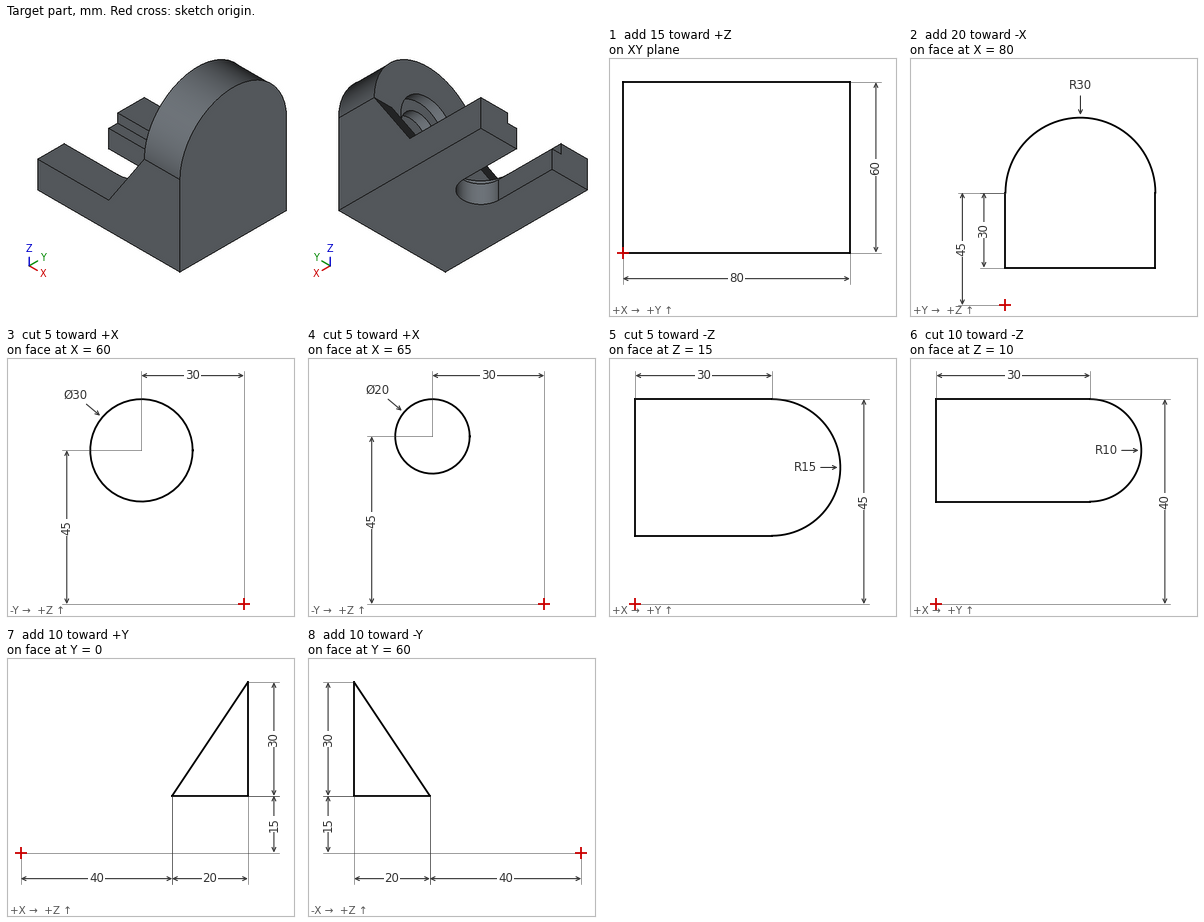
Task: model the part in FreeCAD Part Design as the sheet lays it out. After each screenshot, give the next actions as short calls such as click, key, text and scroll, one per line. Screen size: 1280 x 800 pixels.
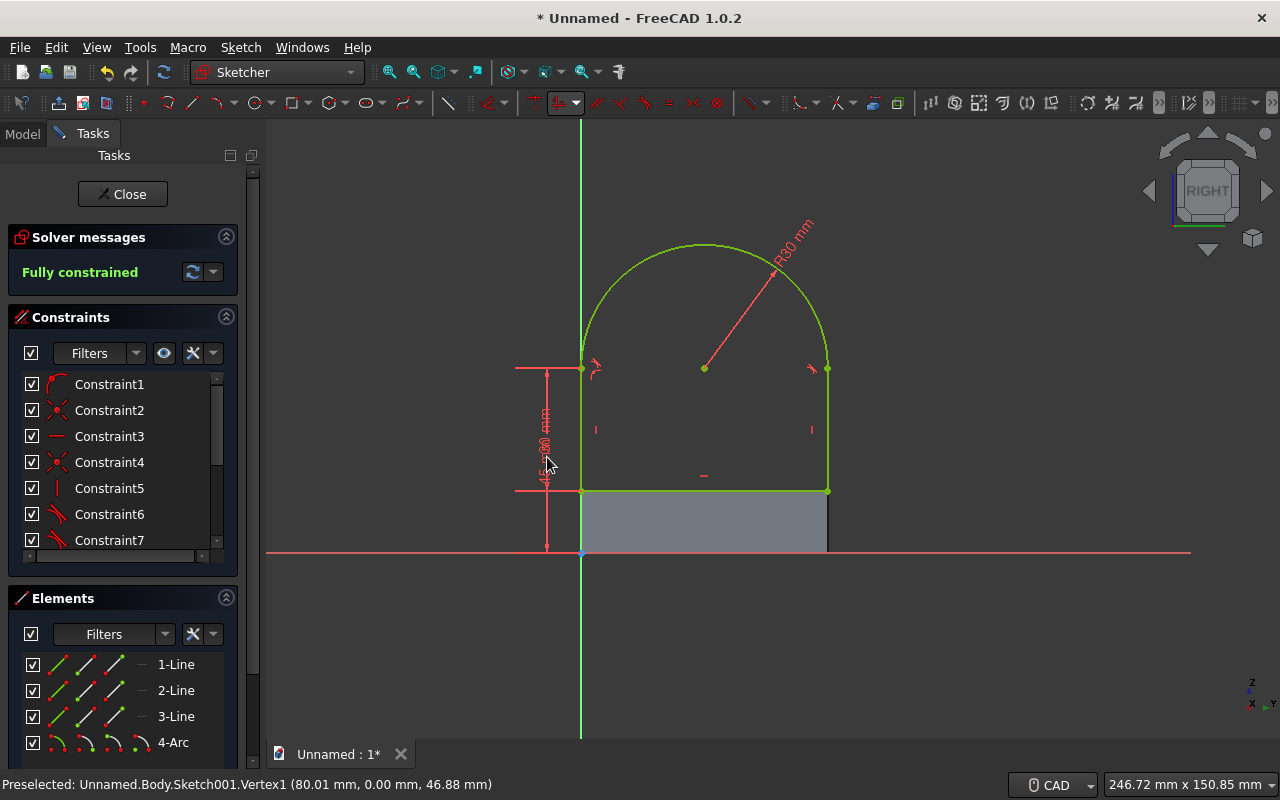
click(123, 194)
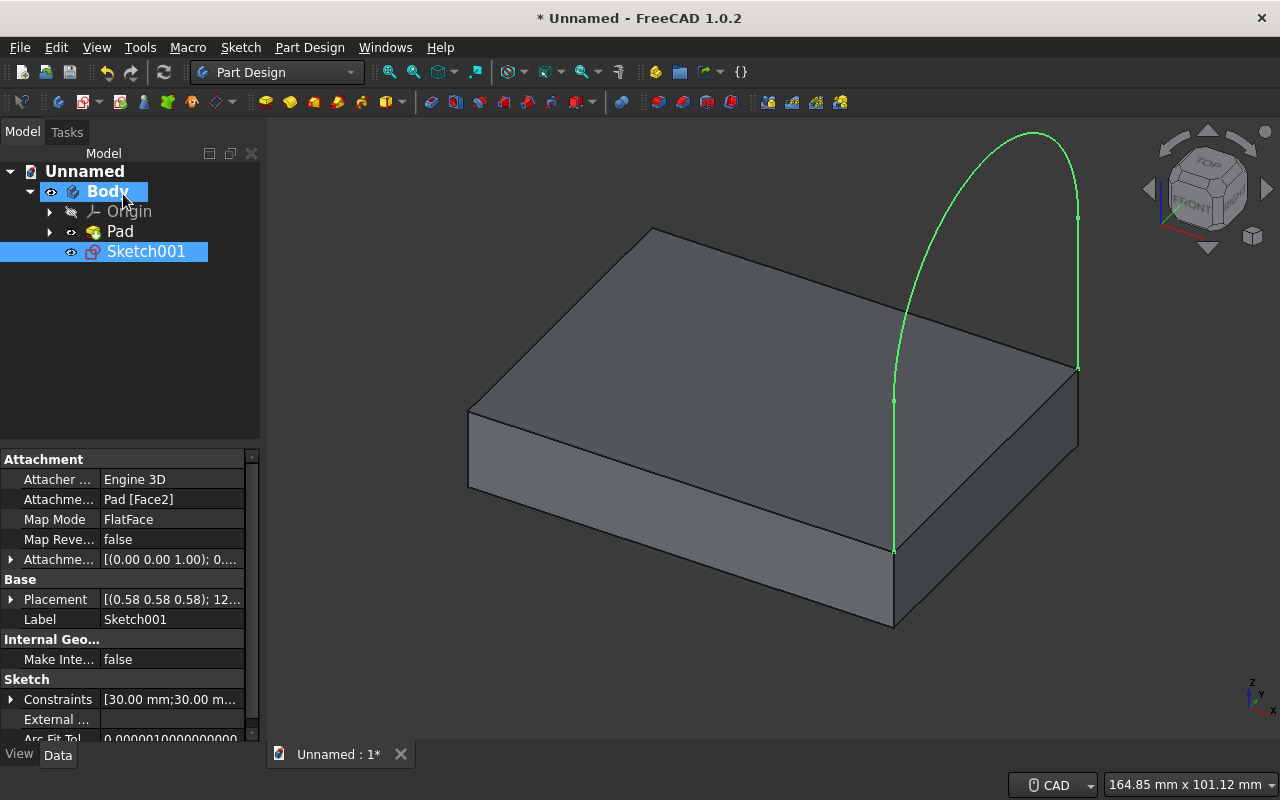
click(266, 102)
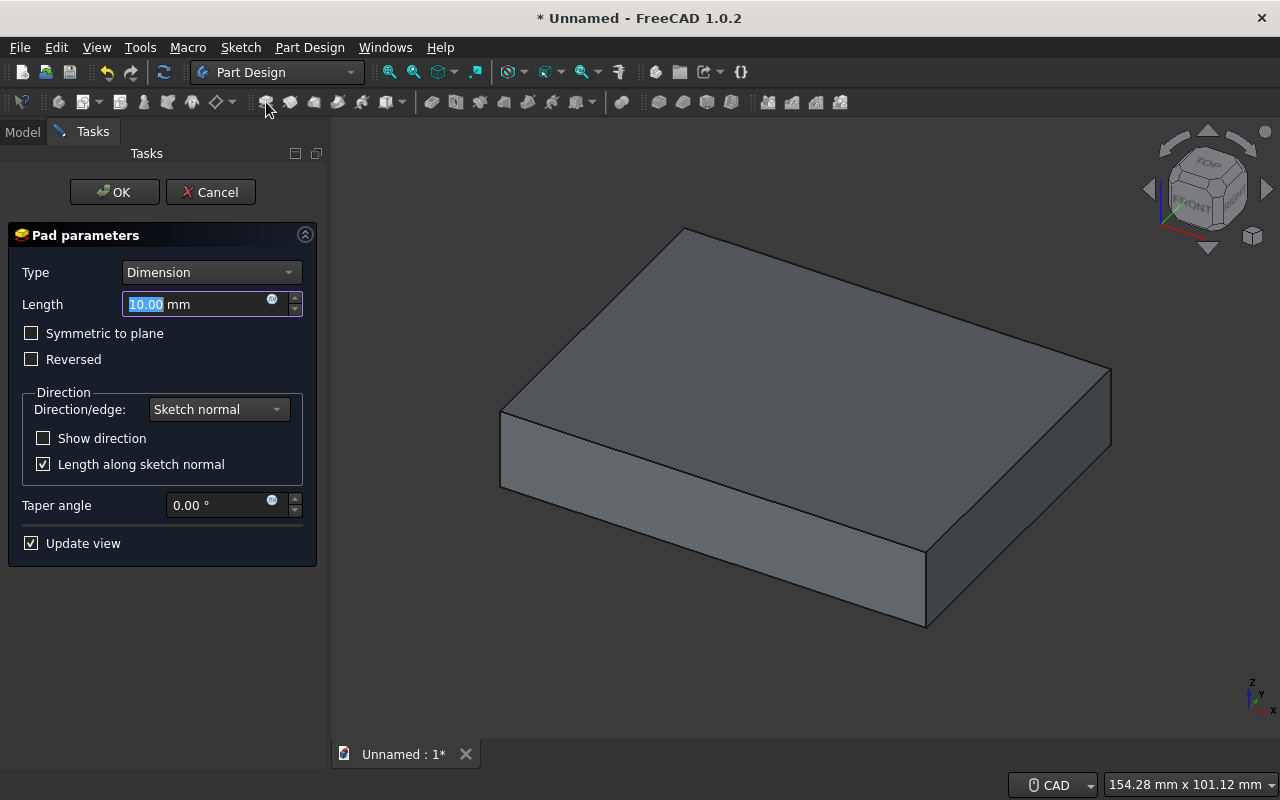
text(20)
key(Tab)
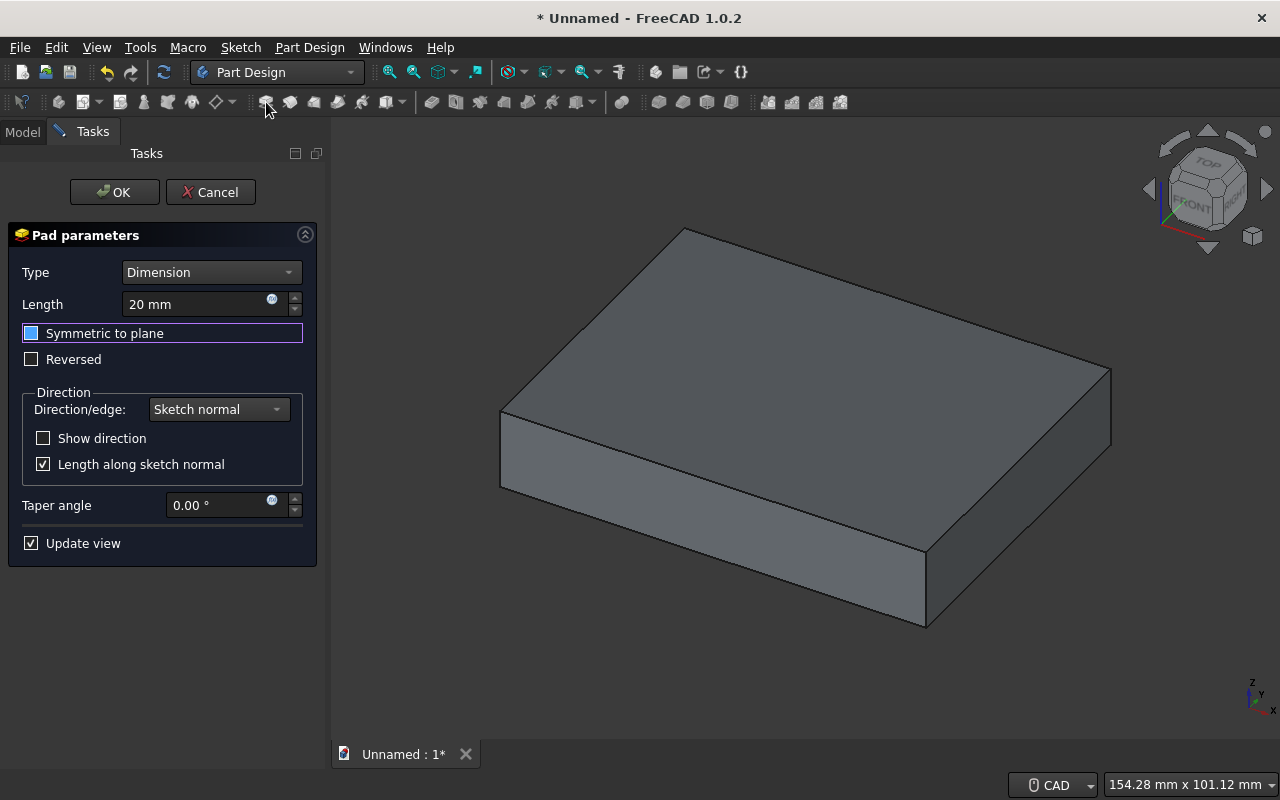
click(30, 359)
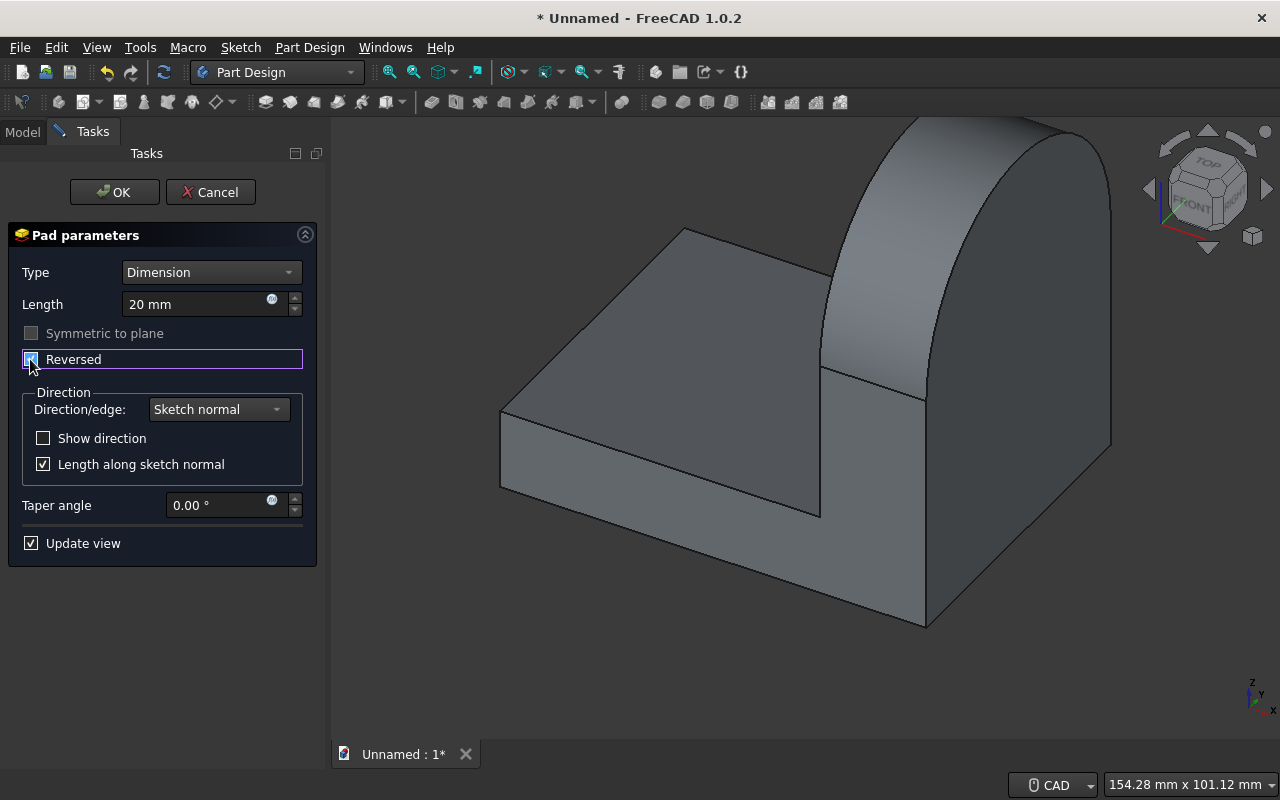
click(115, 192)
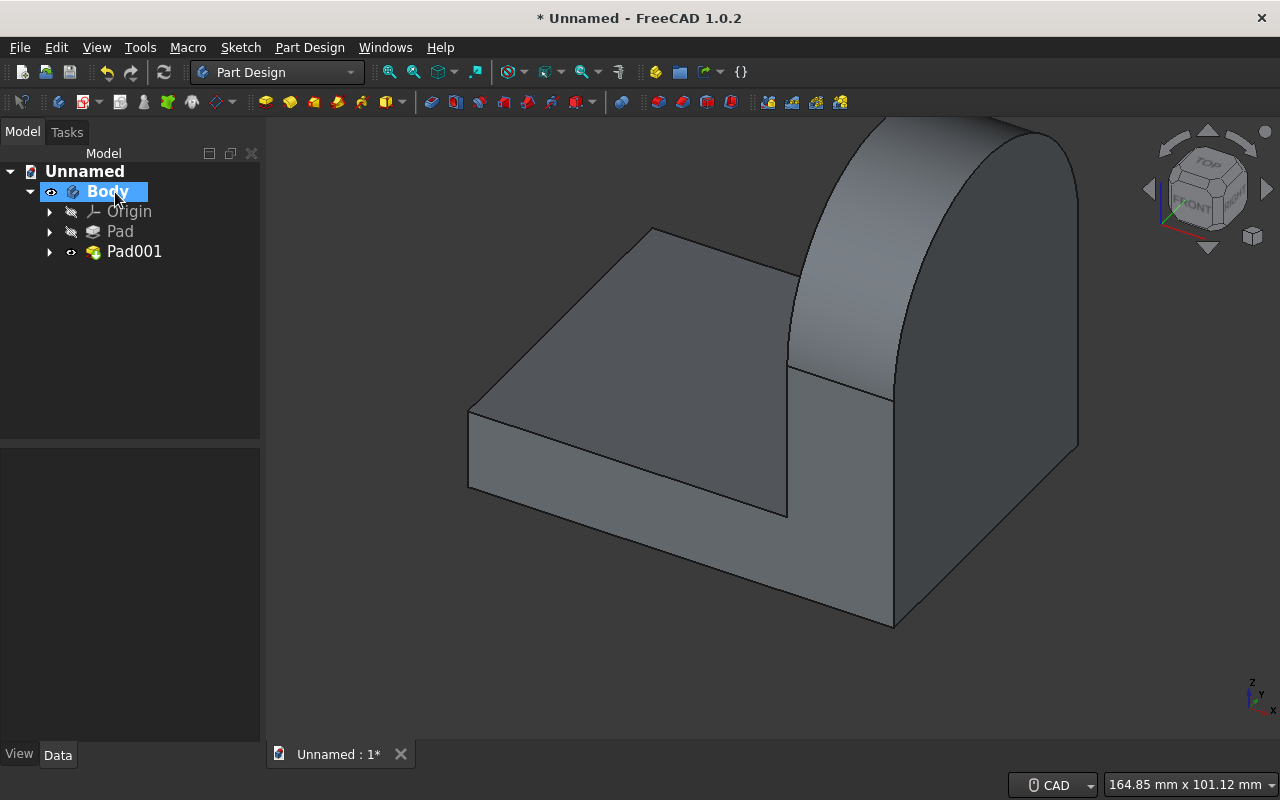
click(390, 72)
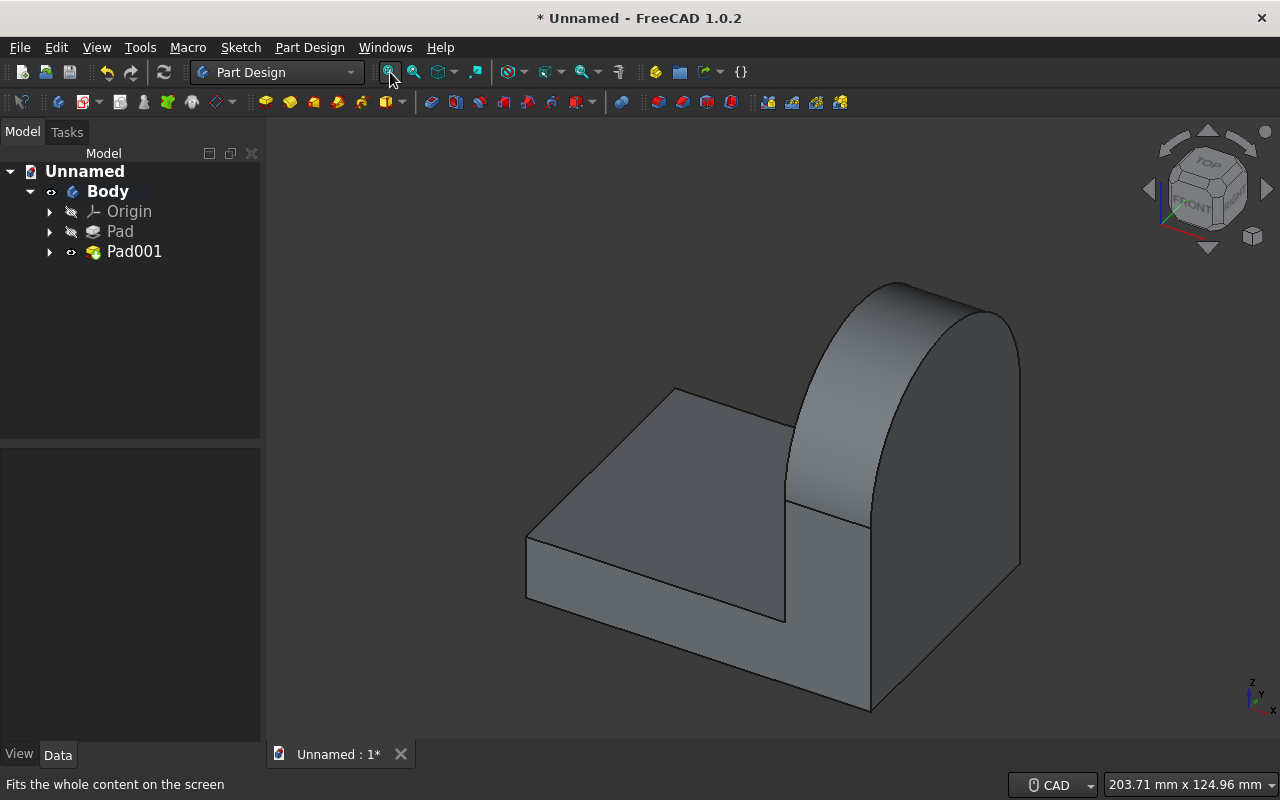
key(6)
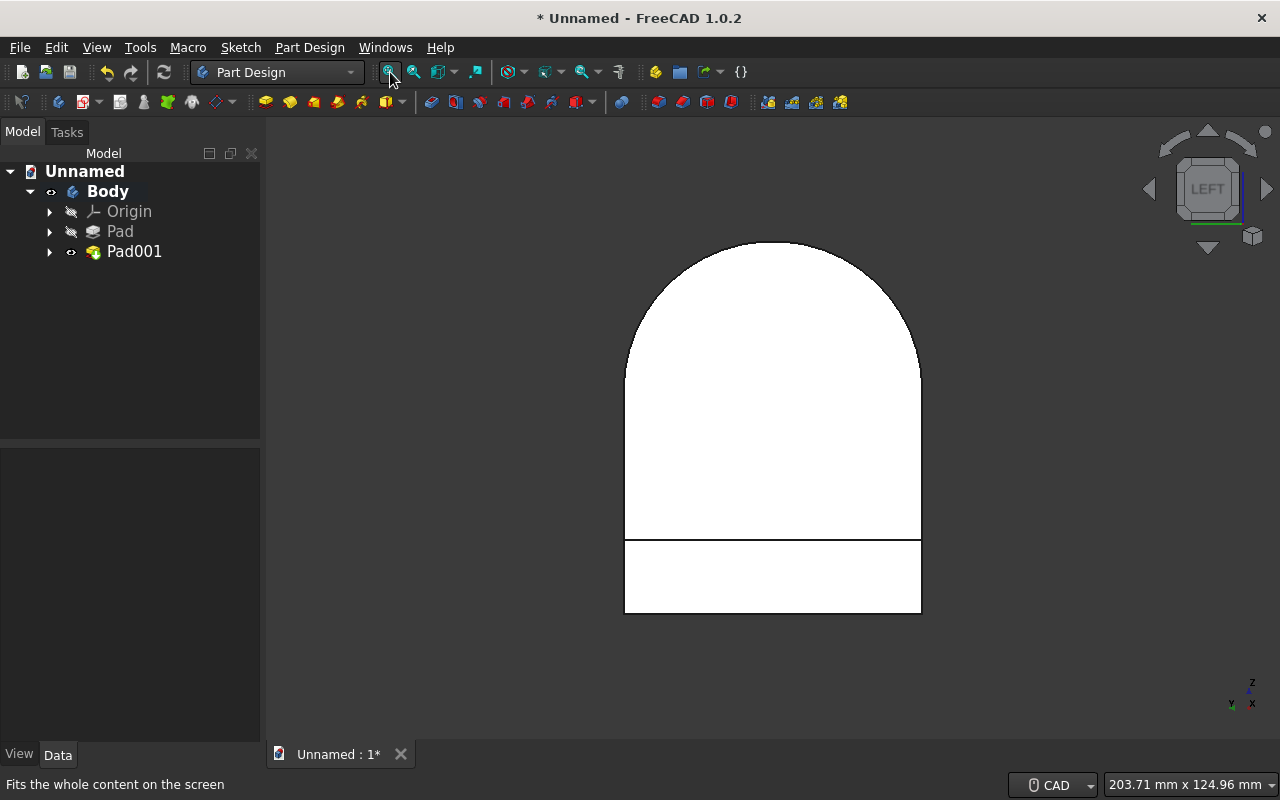
click(773, 389)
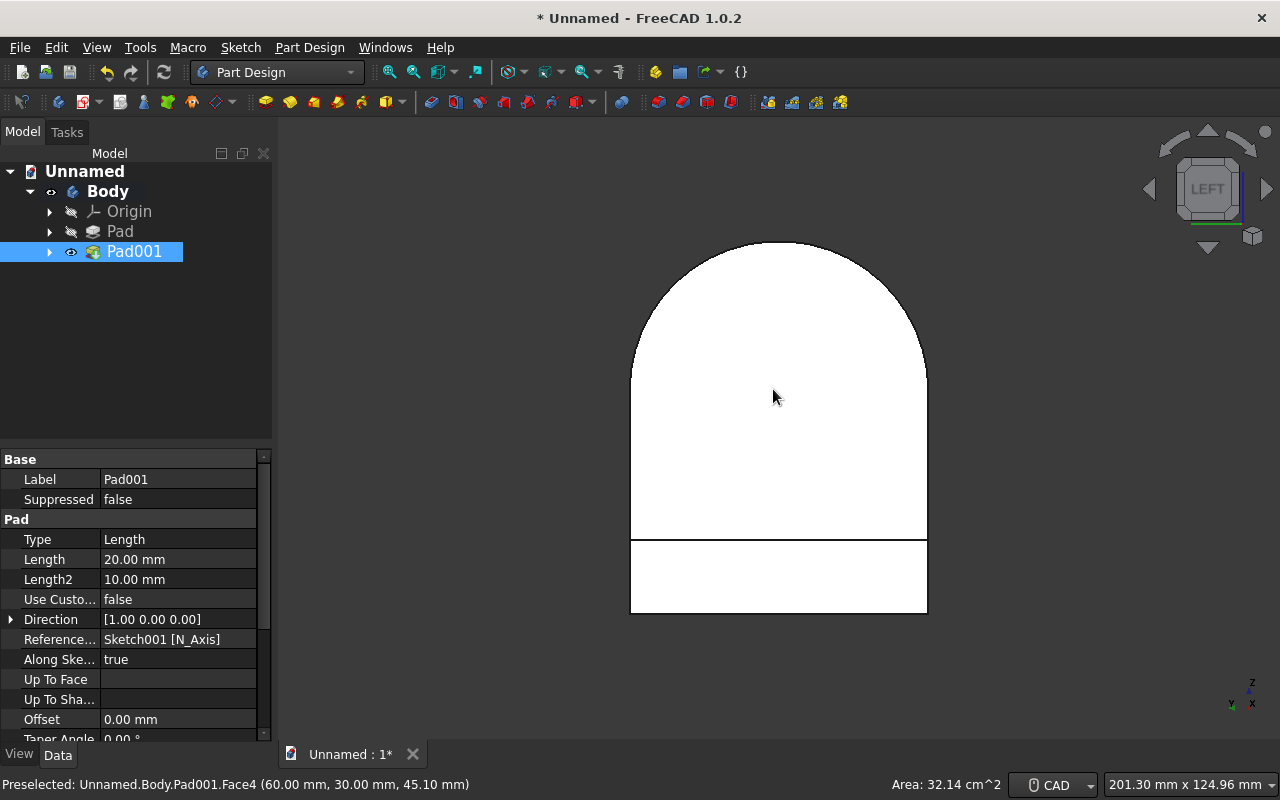
click(84, 102)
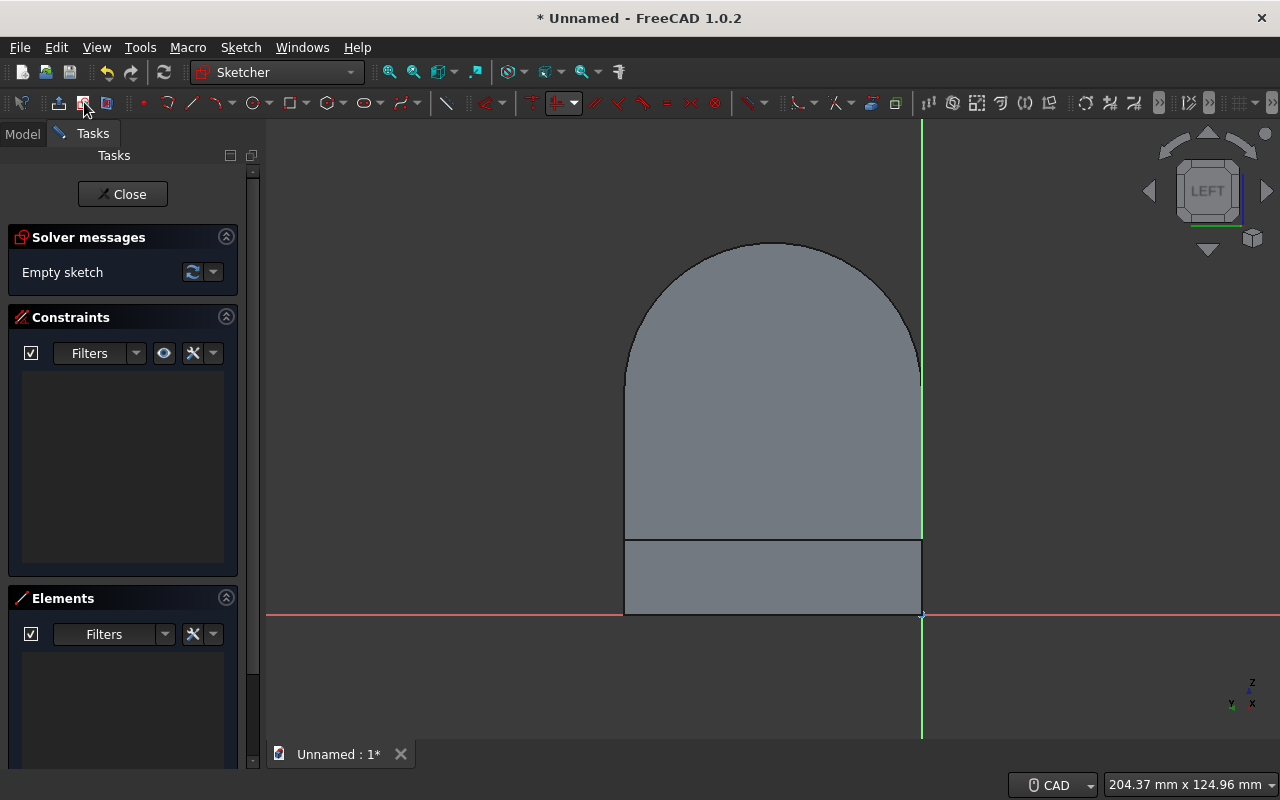
click(254, 104)